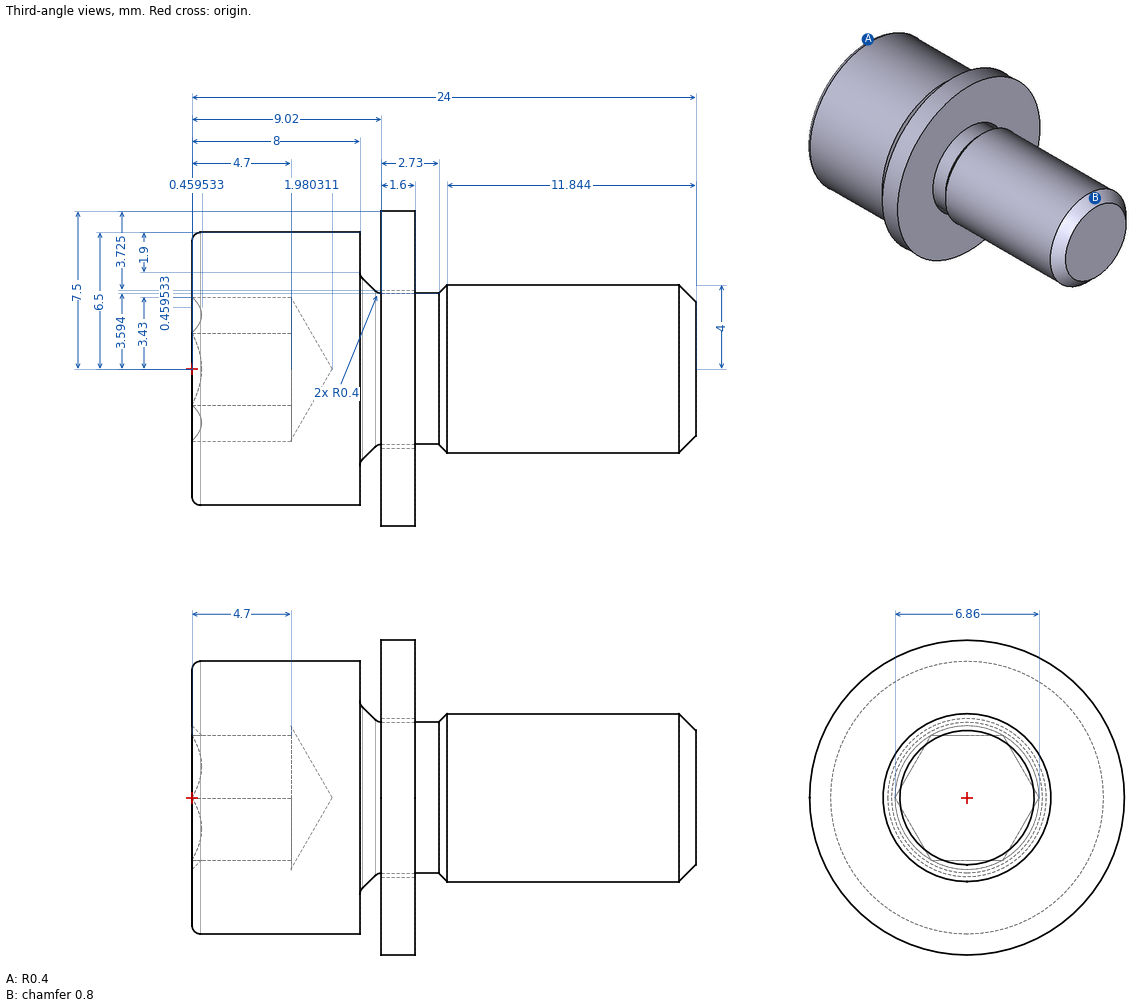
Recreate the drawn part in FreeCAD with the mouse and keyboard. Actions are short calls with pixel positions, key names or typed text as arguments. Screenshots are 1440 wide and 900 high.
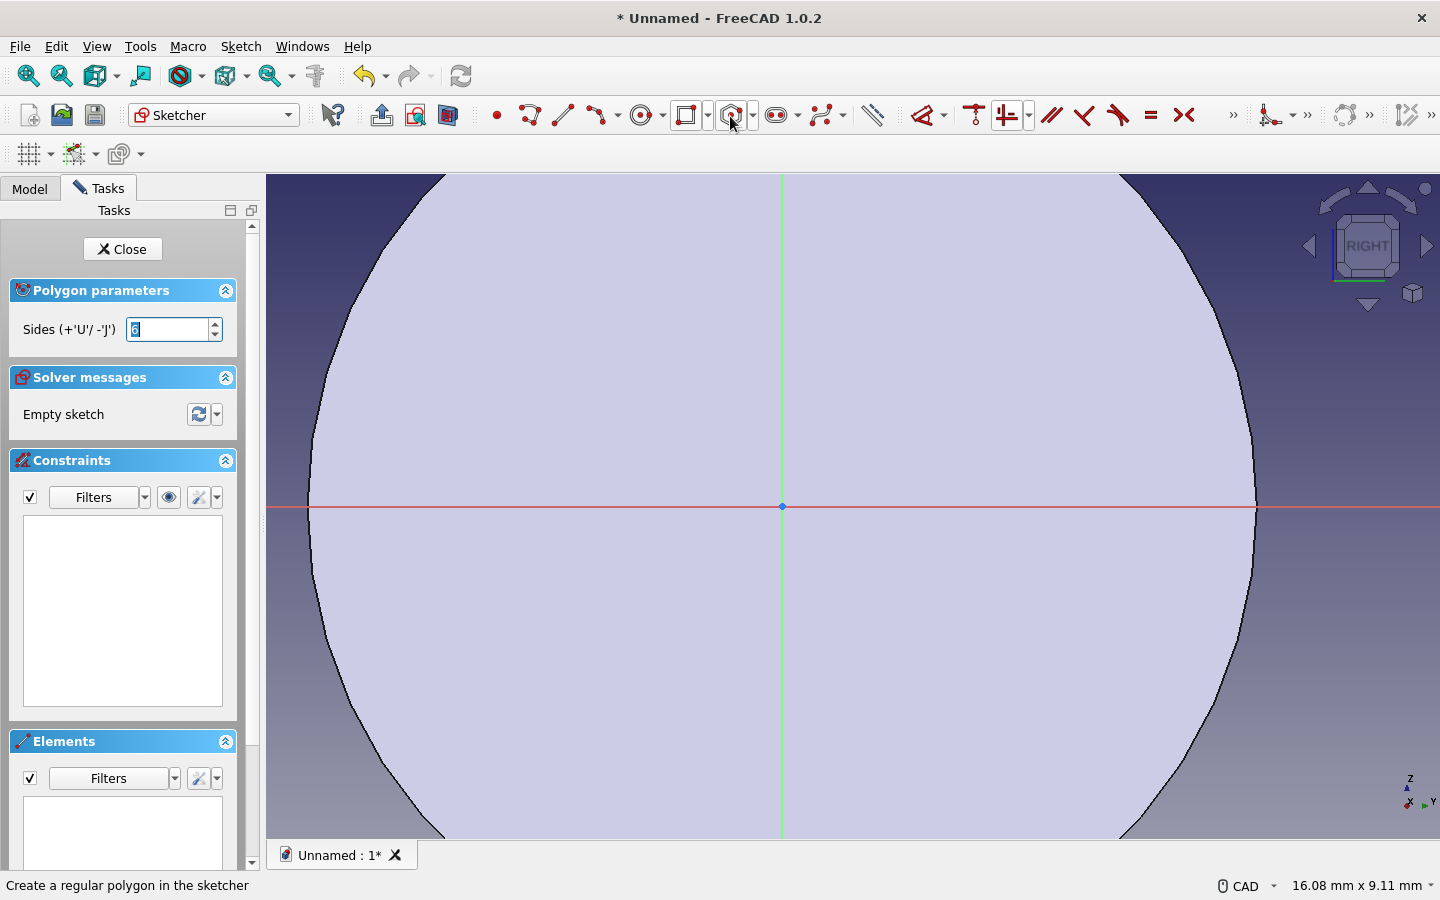
click(782, 506)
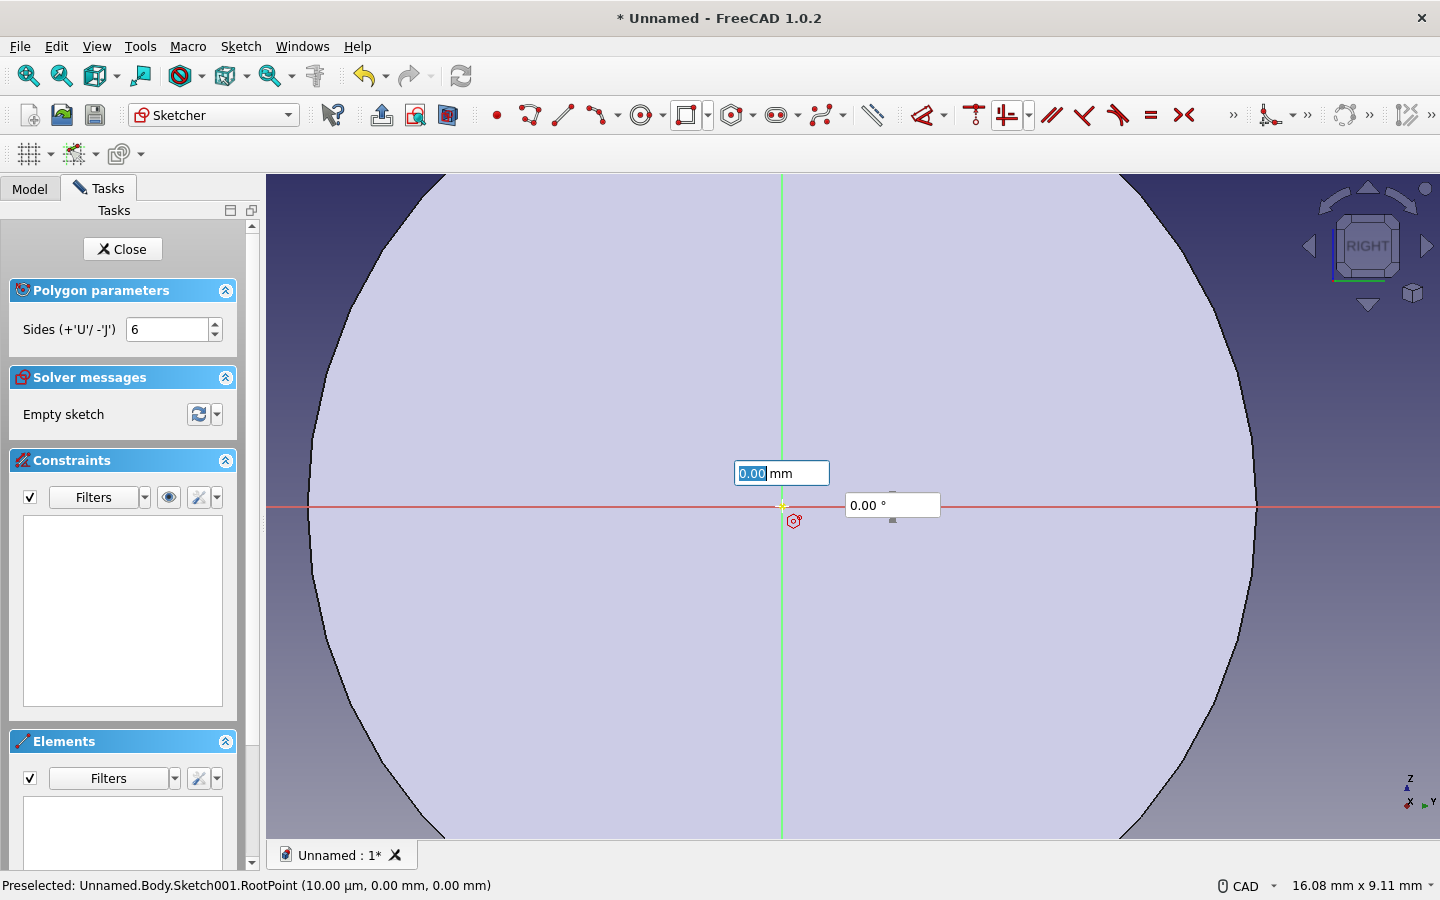
click(1033, 506)
right_click(1033, 506)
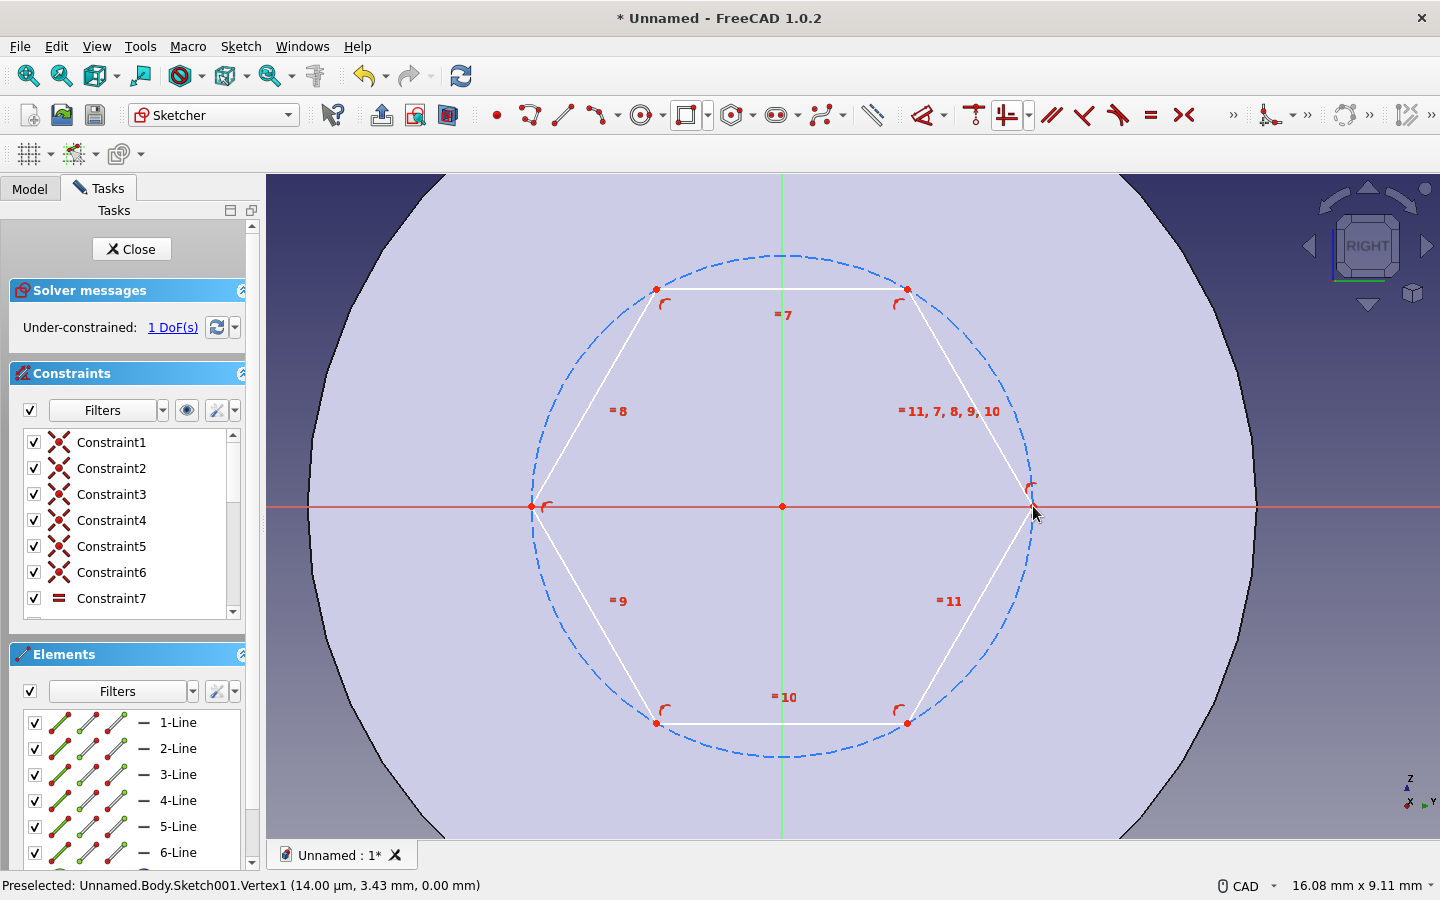
click(922, 116)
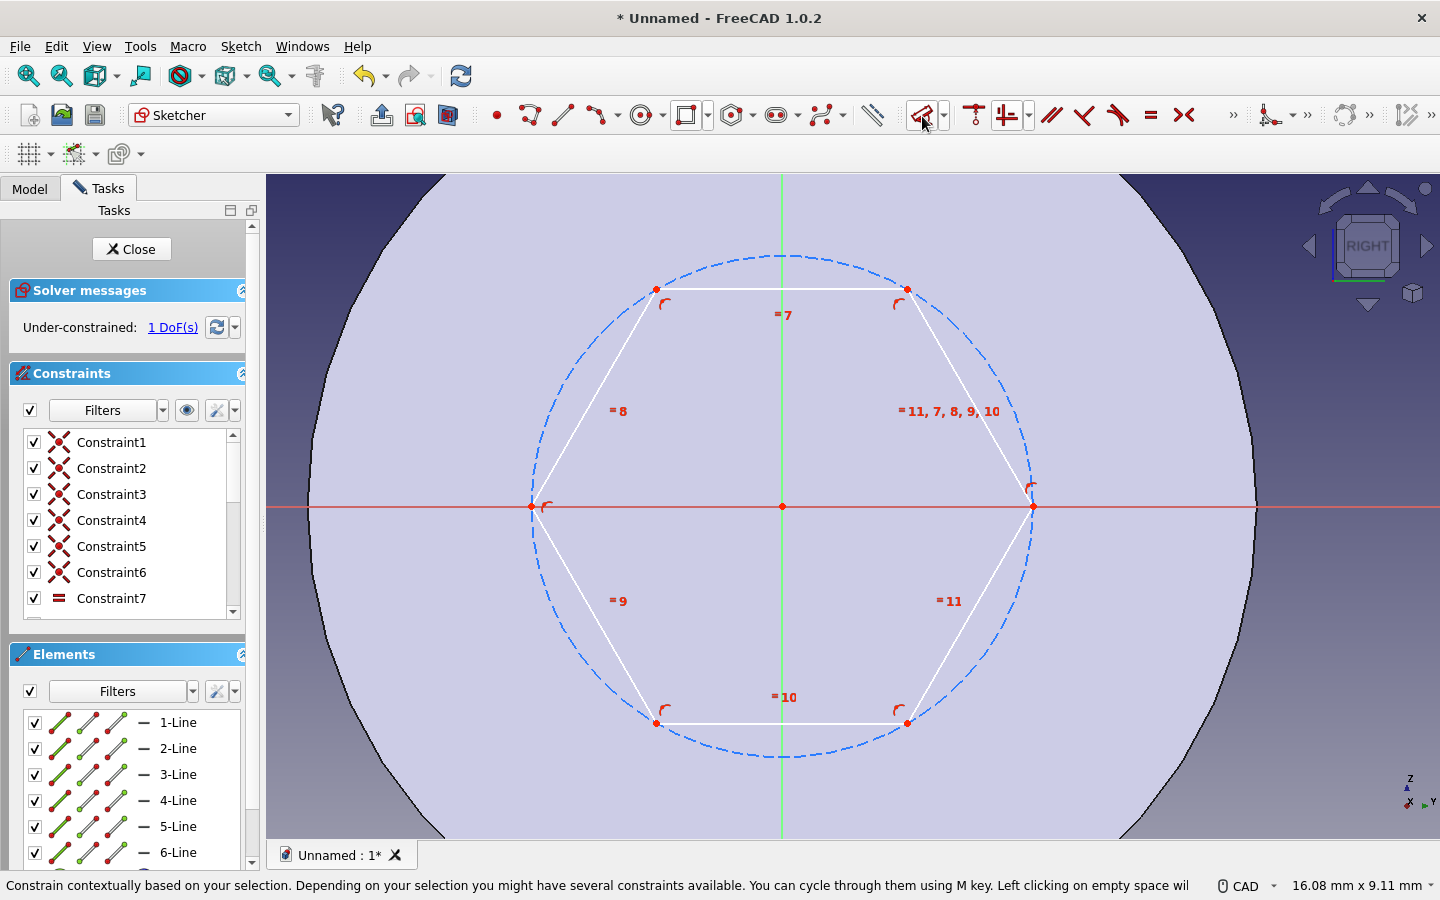
click(531, 506)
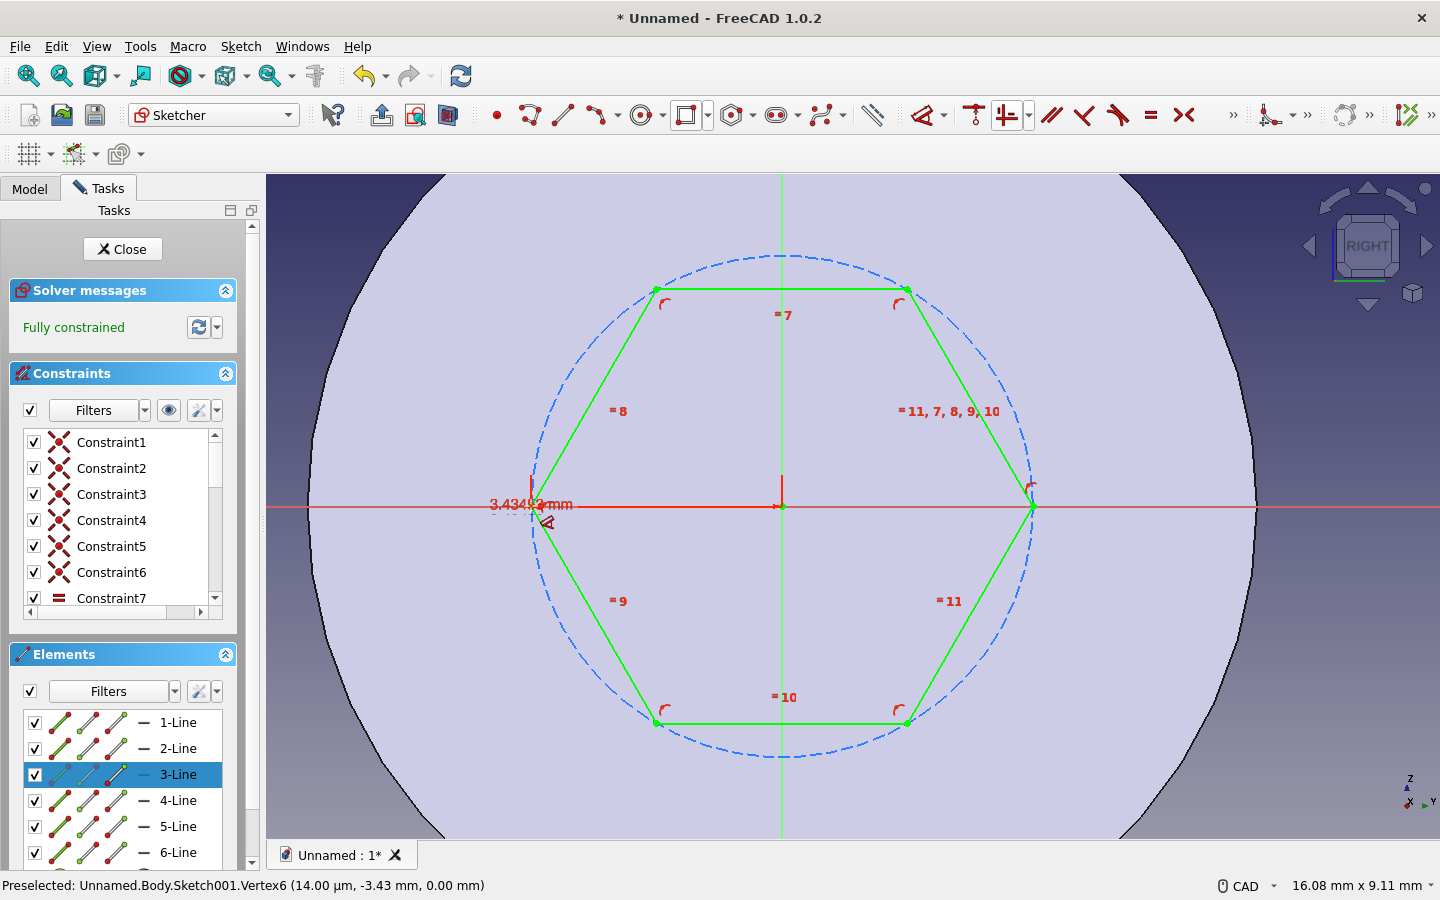
click(1033, 506)
click(667, 540)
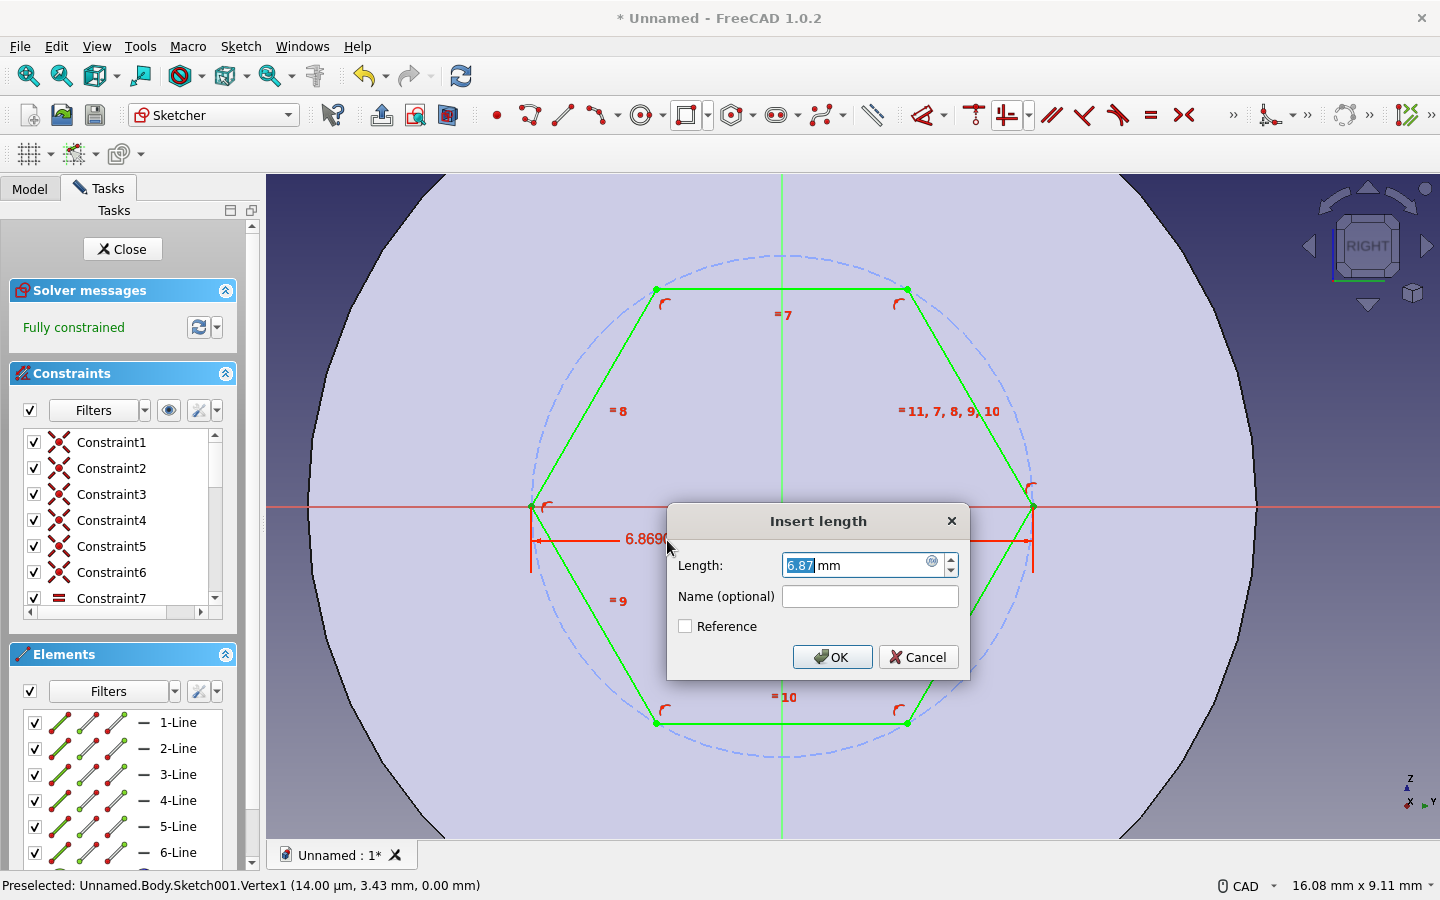
text(6.86)
key(Return)
key(Escape)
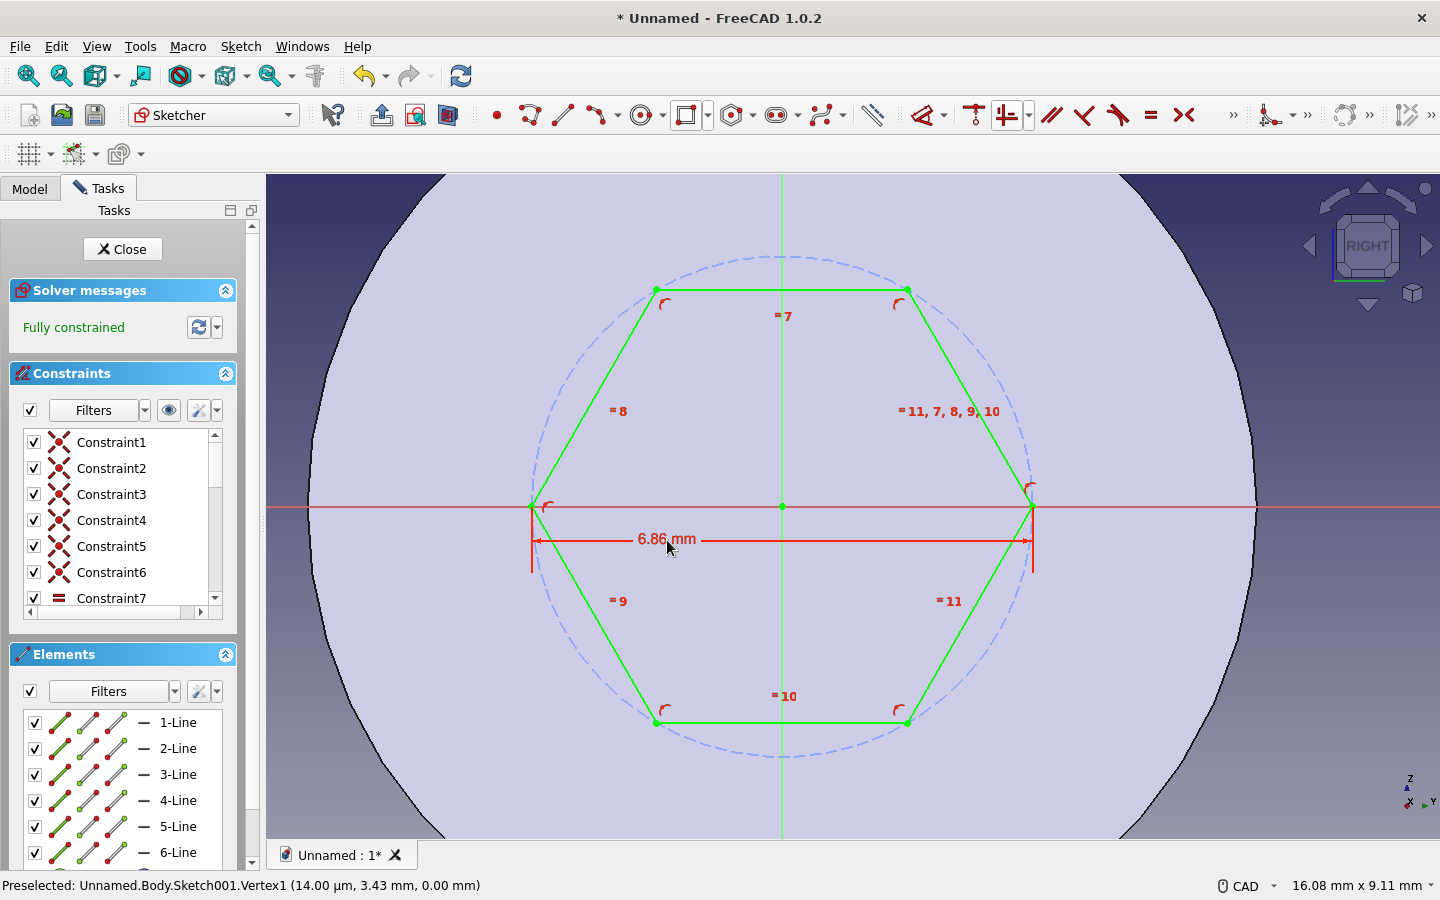
click(123, 249)